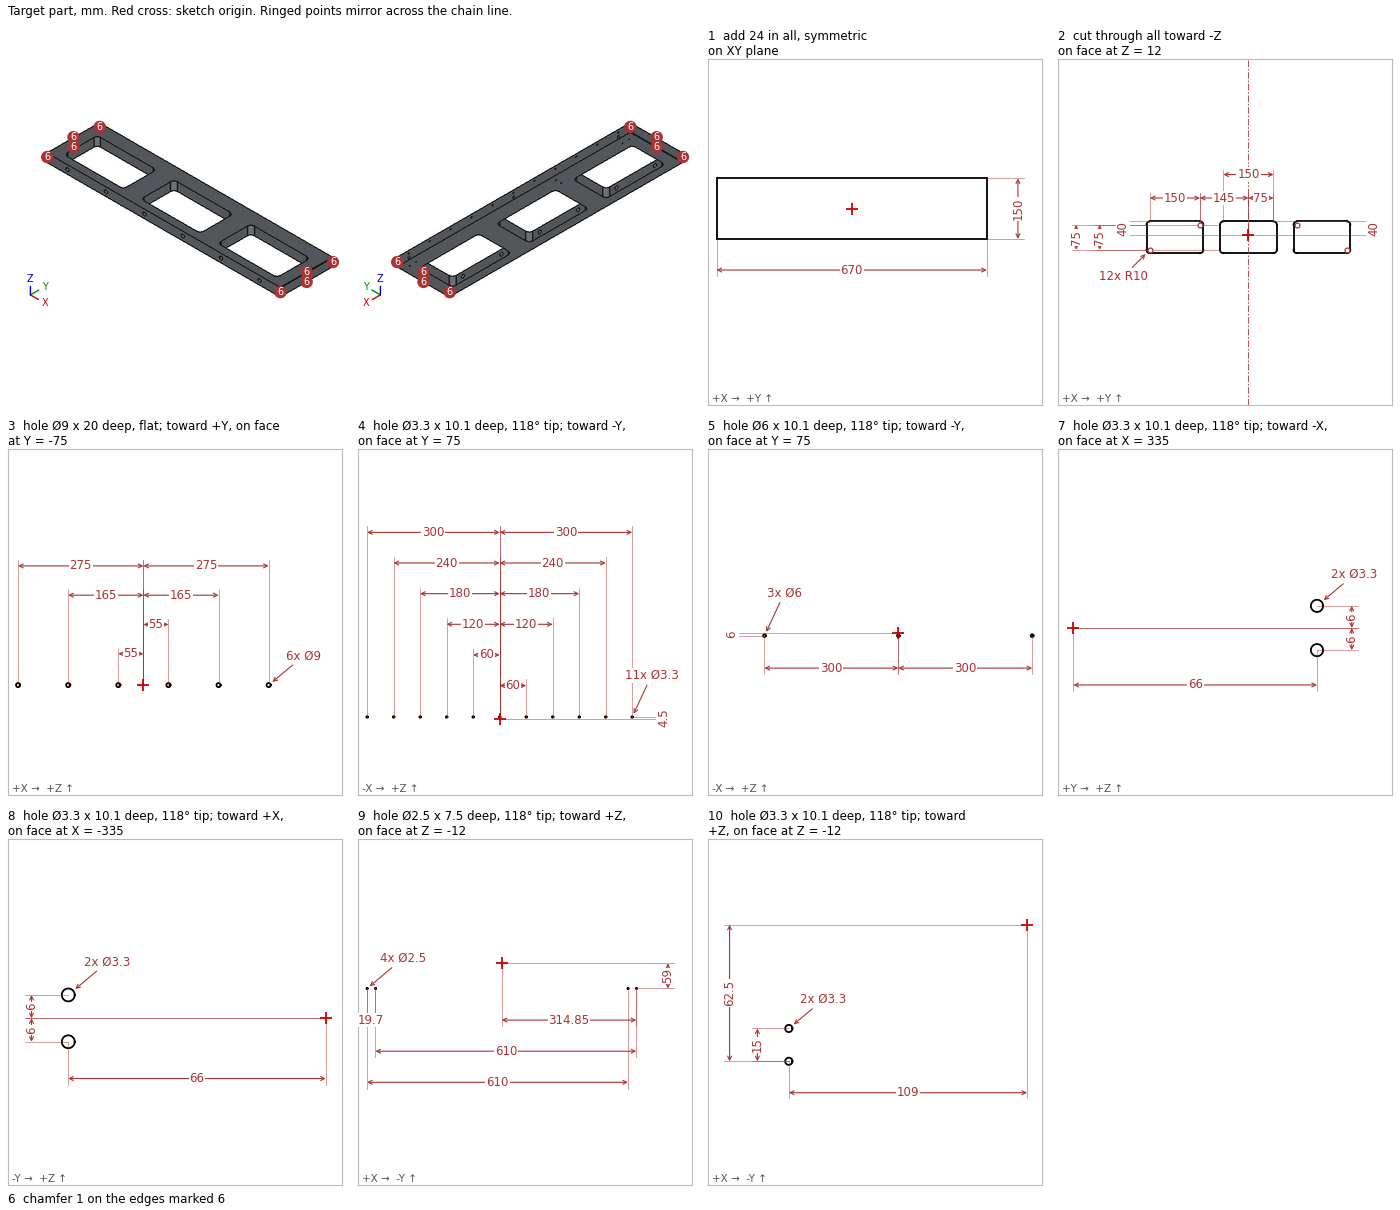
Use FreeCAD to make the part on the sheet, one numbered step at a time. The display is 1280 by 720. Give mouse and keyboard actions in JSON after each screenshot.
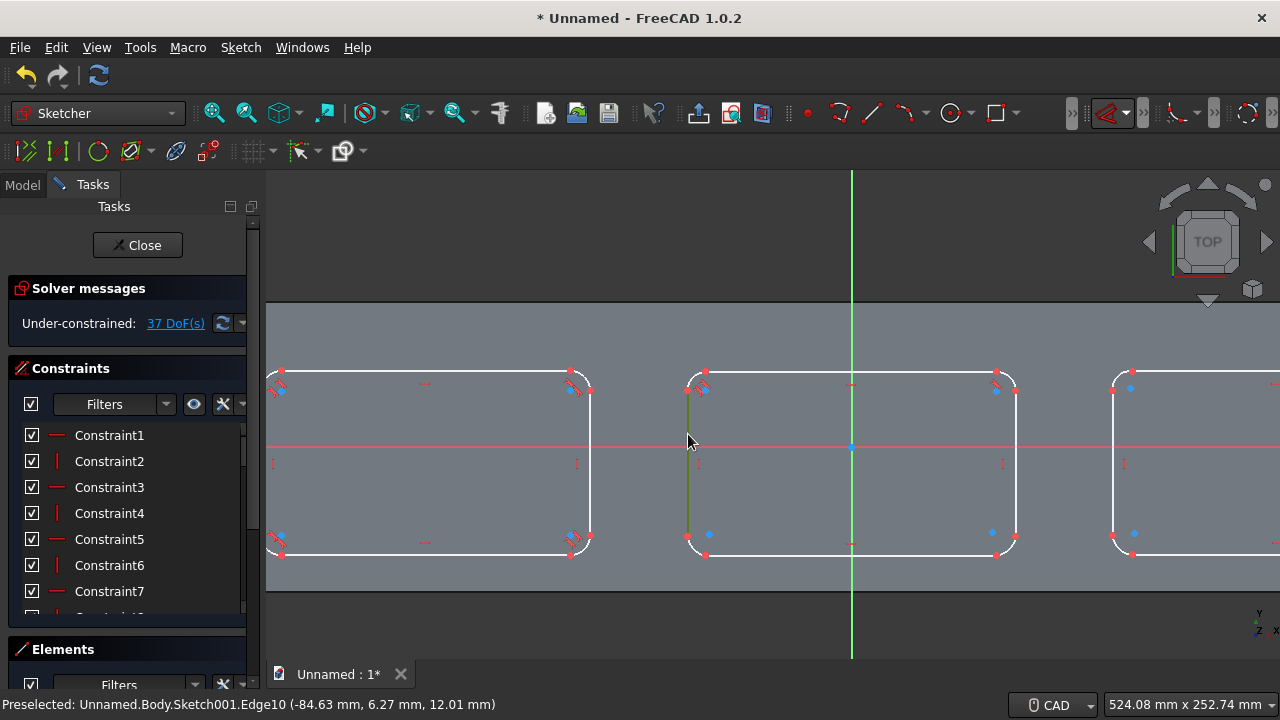
{"action": "left_click", "coordinate": [694, 549]}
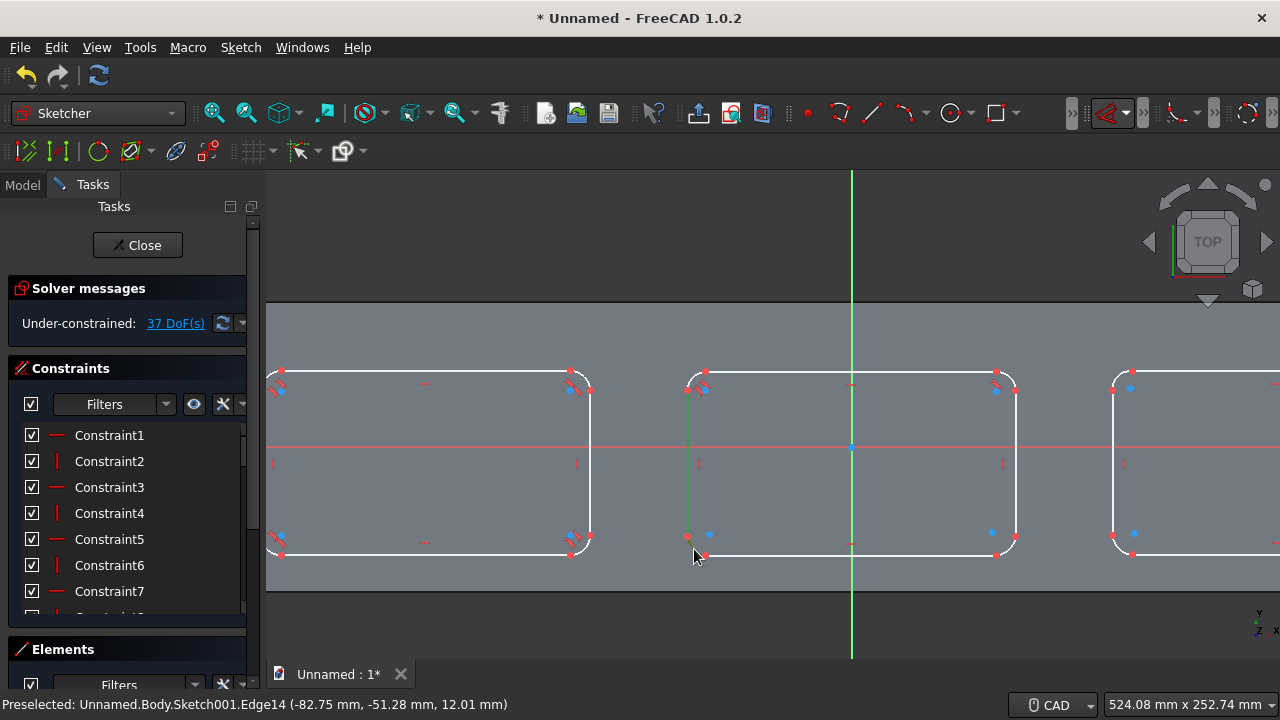
{"action": "key", "text": "t"}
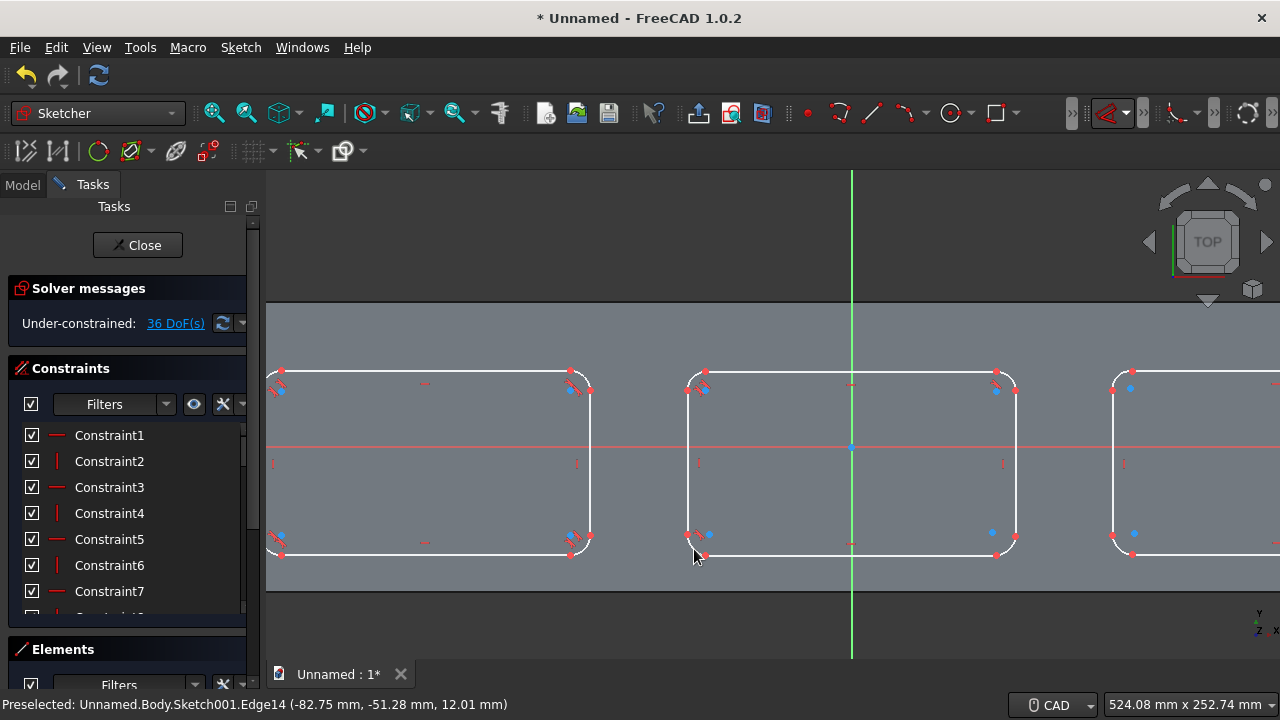
{"action": "left_click", "coordinate": [793, 556]}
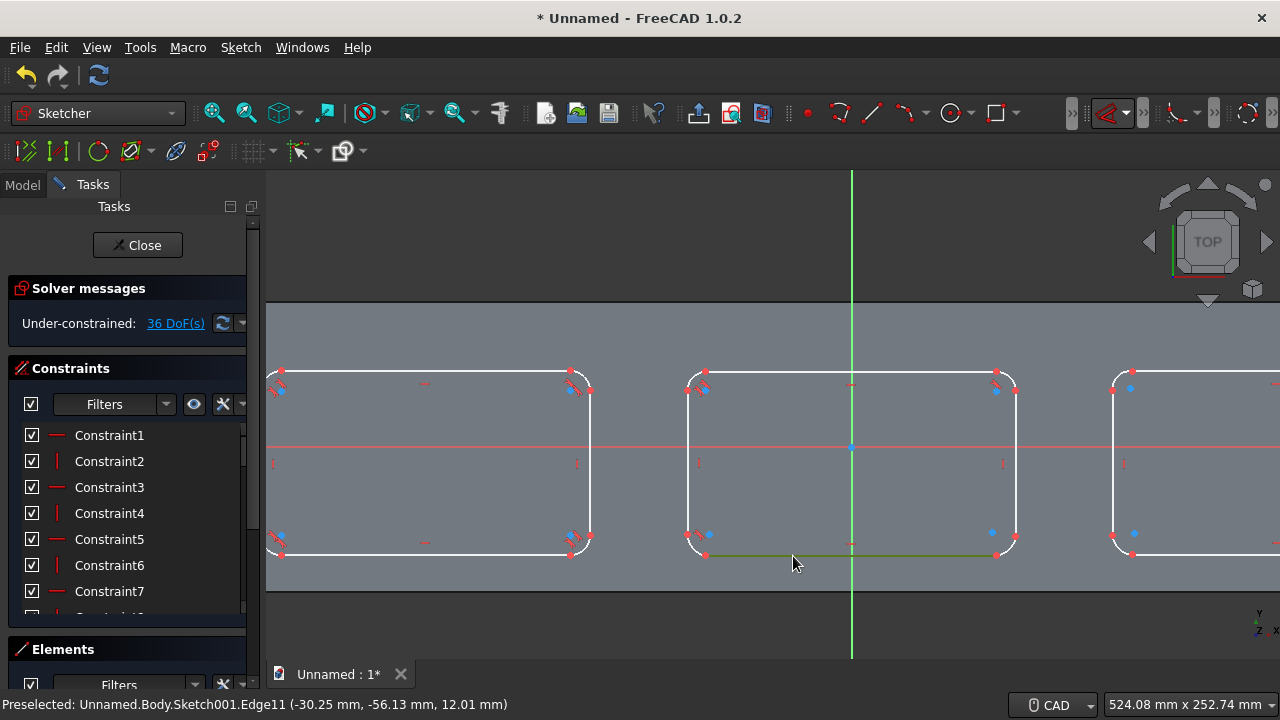
{"action": "scroll", "coordinate": [690, 543], "scroll_direction": "up", "scroll_amount": 3}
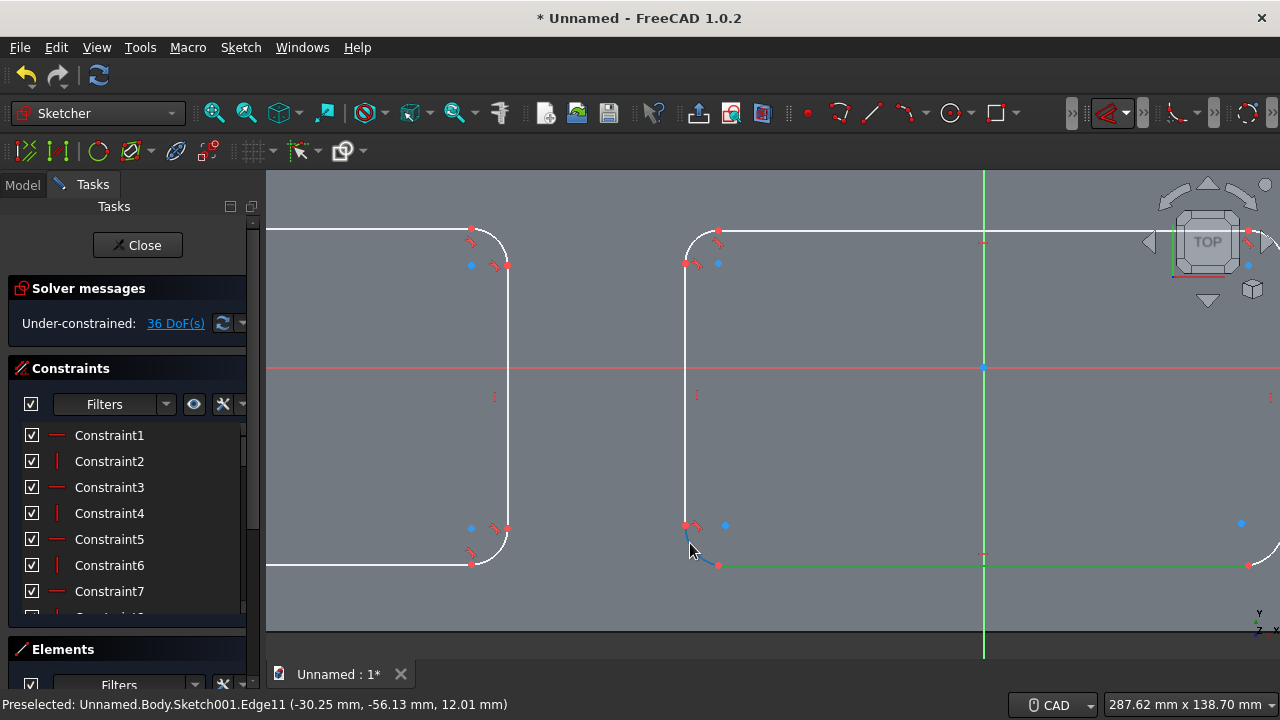
{"action": "left_click", "coordinate": [689, 542]}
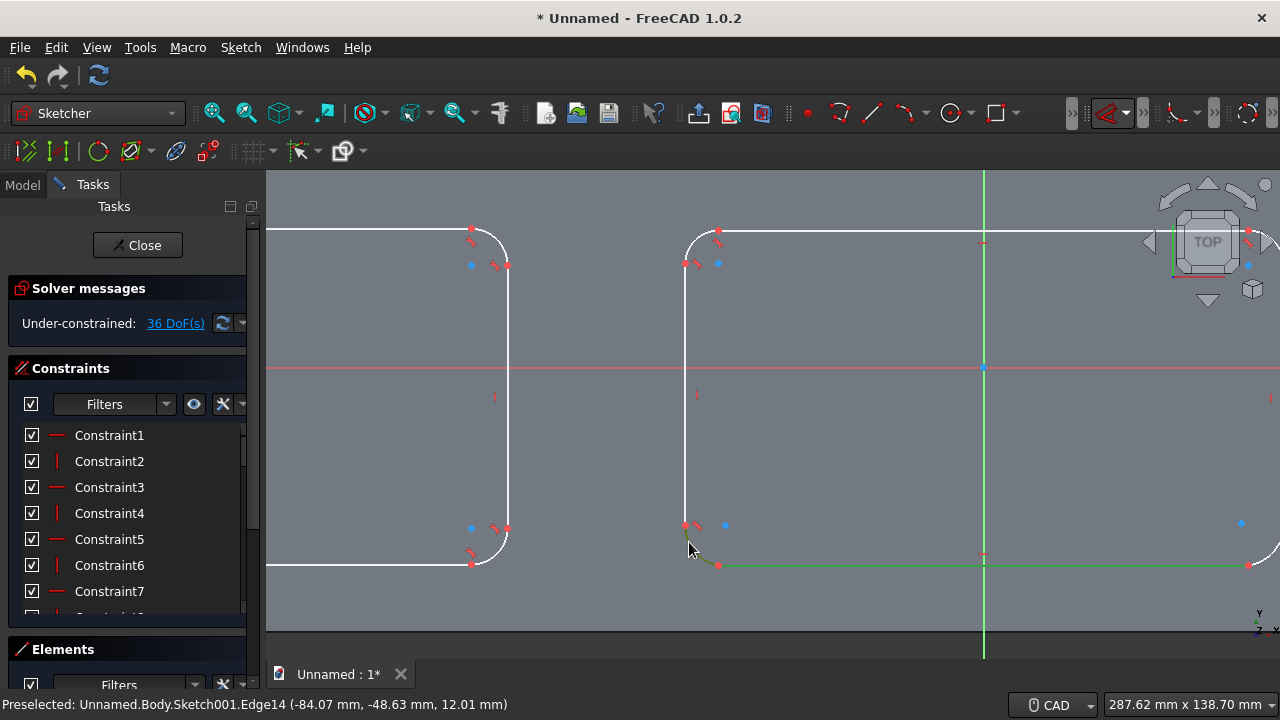
{"action": "key", "text": "t"}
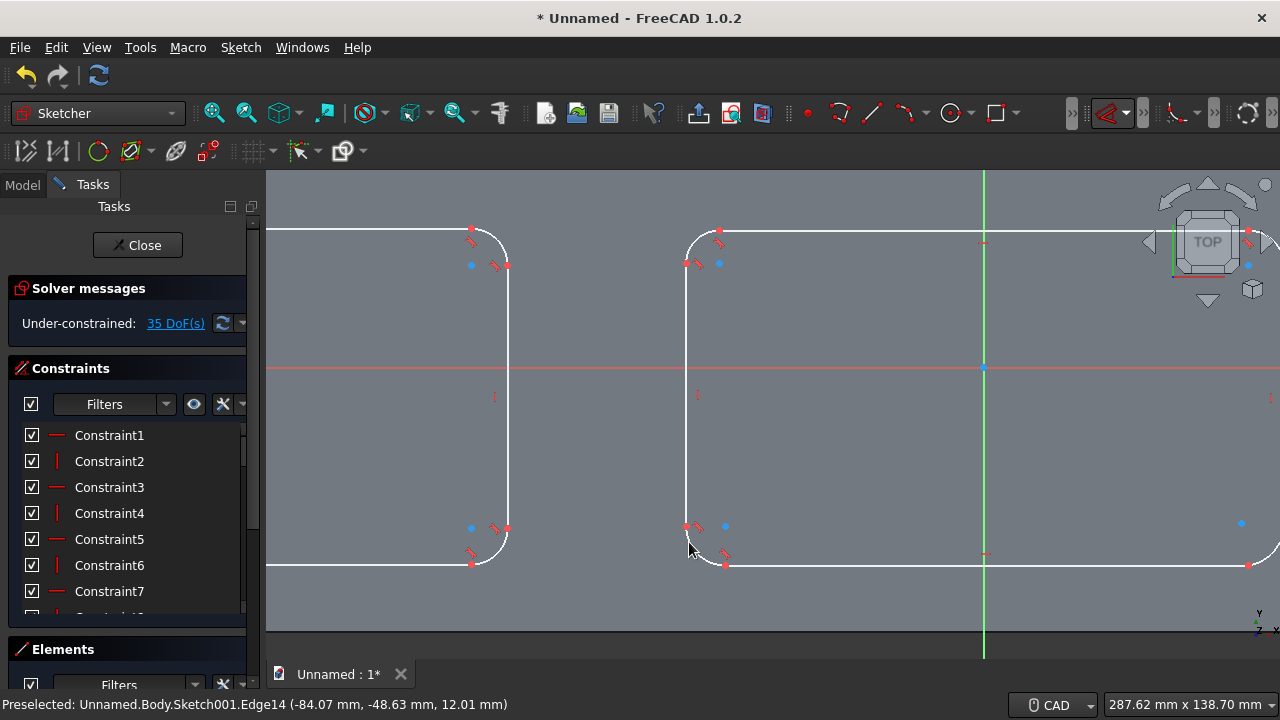
{"action": "scroll", "coordinate": [613, 421], "scroll_direction": "down", "scroll_amount": 7}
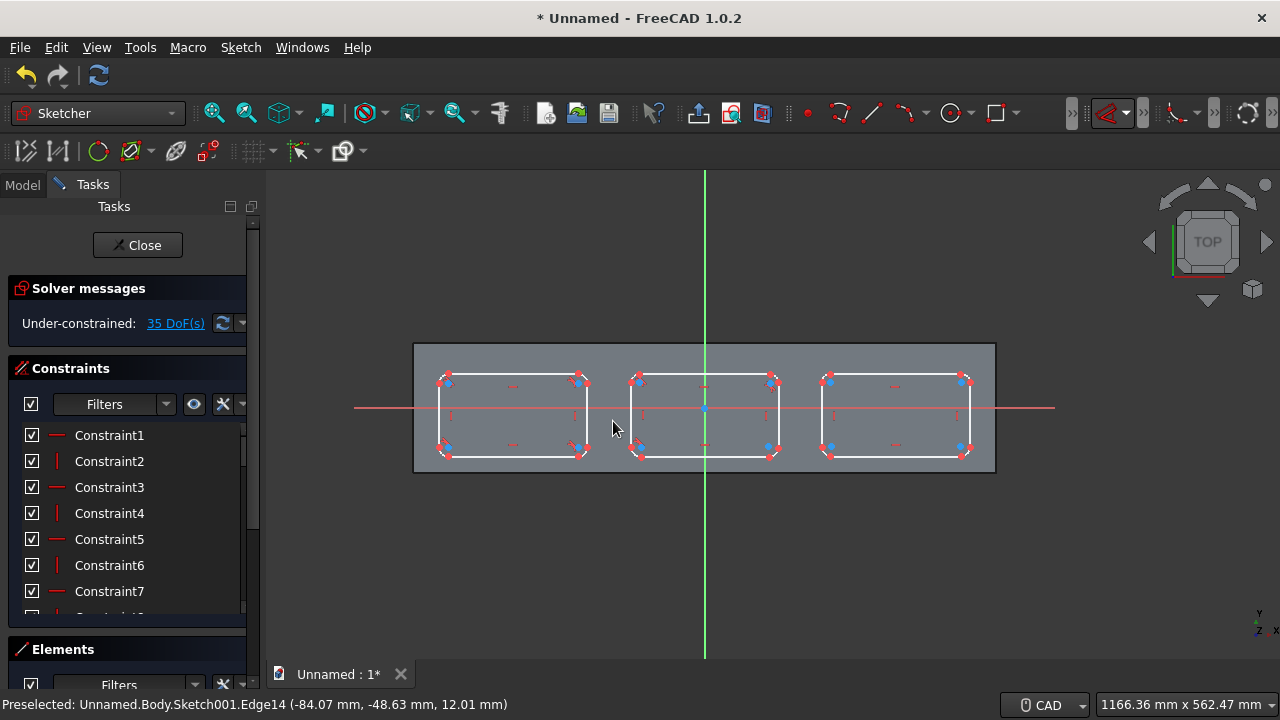
{"action": "left_click", "coordinate": [680, 457]}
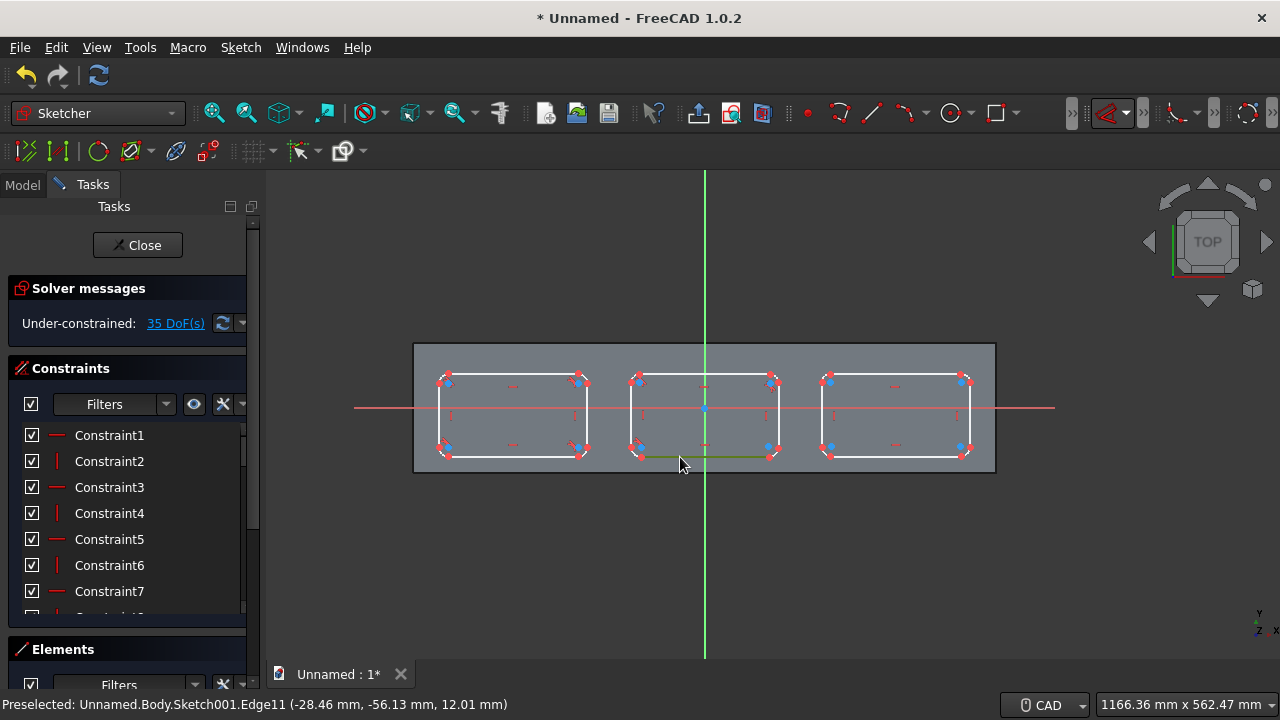
{"action": "scroll", "coordinate": [776, 454], "scroll_direction": "up", "scroll_amount": 4}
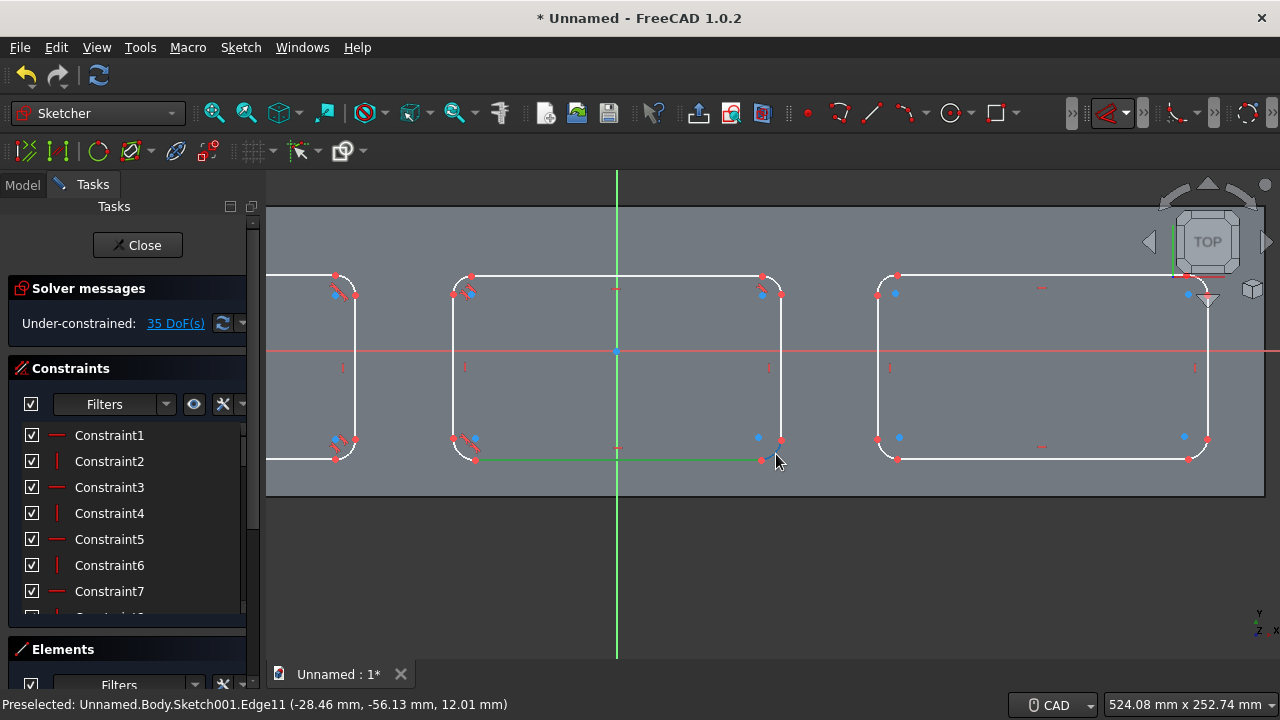
{"action": "left_click", "coordinate": [775, 454]}